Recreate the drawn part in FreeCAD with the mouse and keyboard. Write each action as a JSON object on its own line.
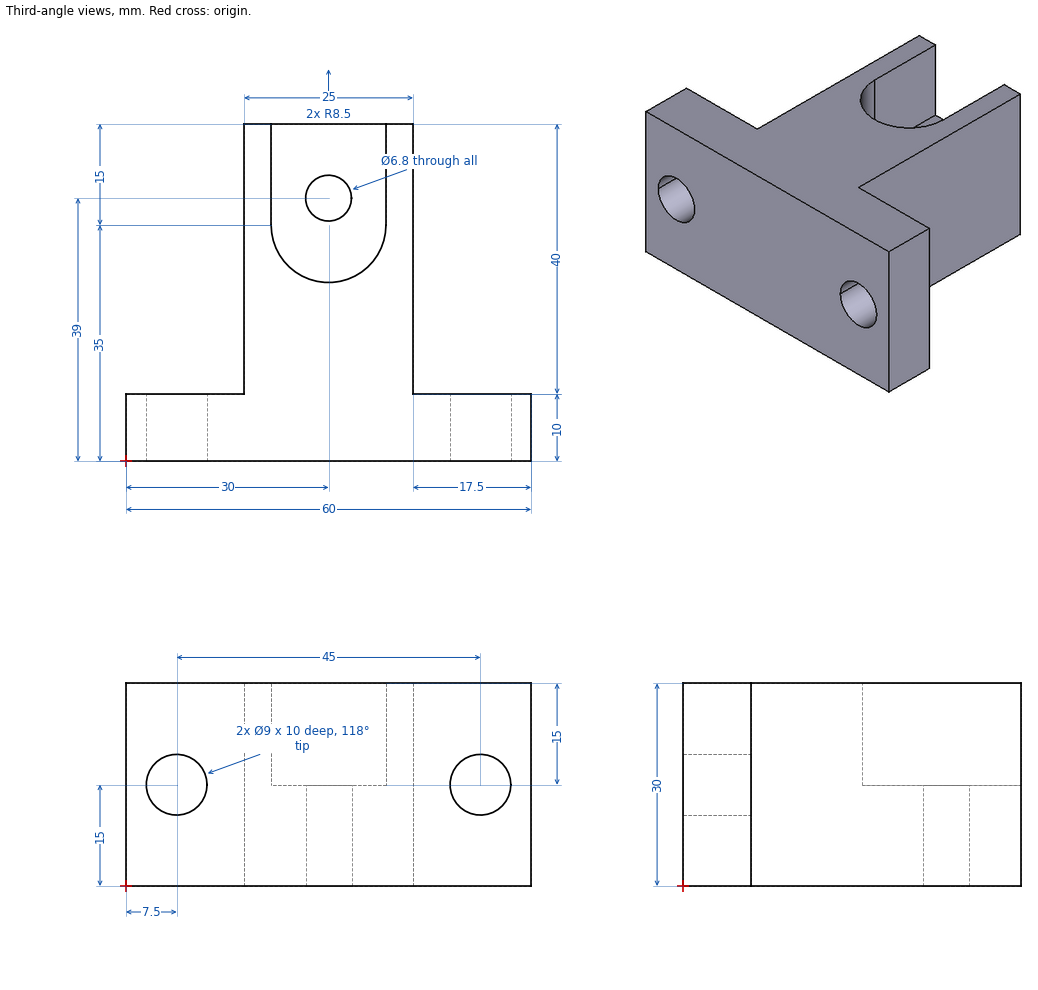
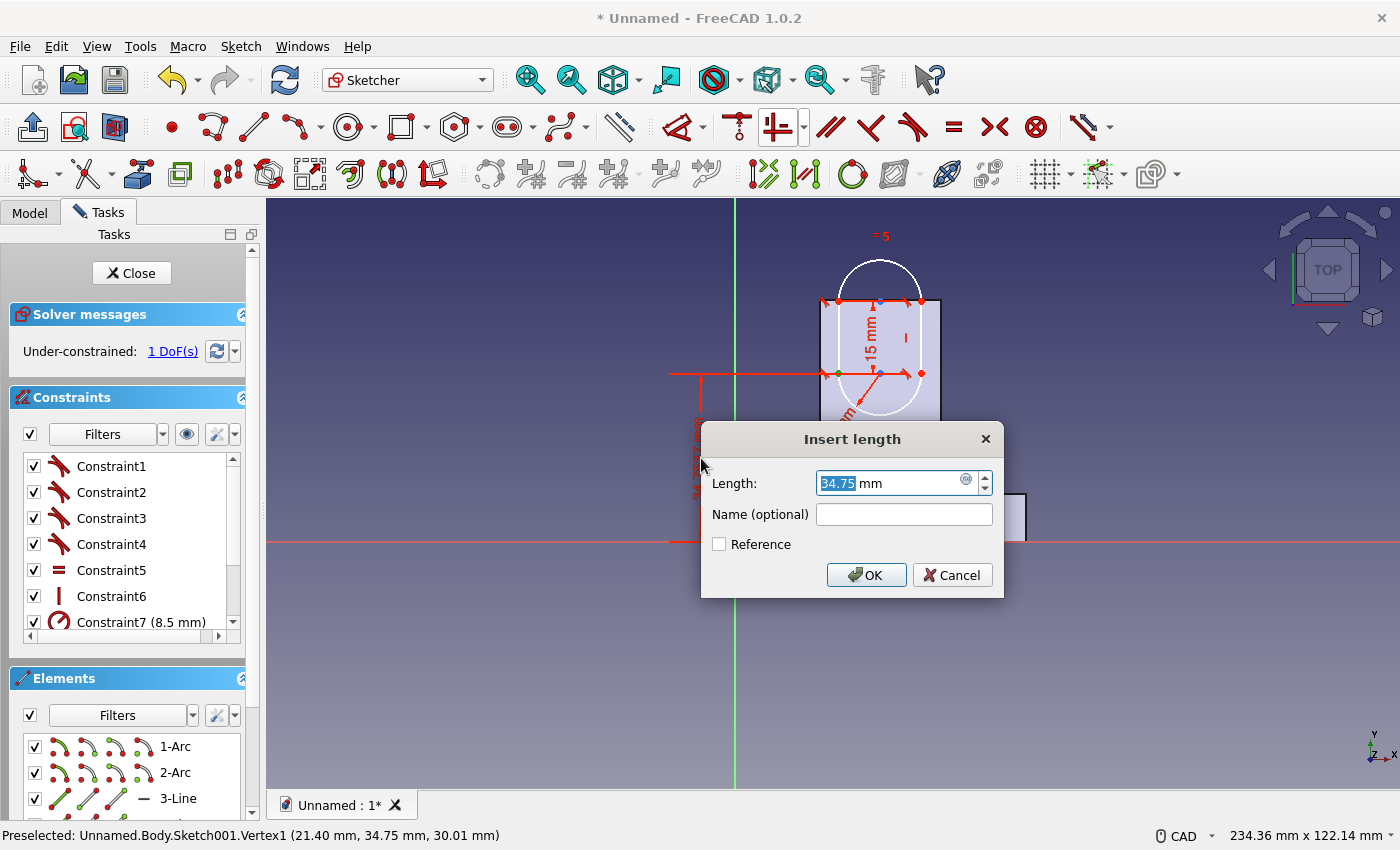
{"action": "type", "text": "35"}
{"action": "key", "text": "Return"}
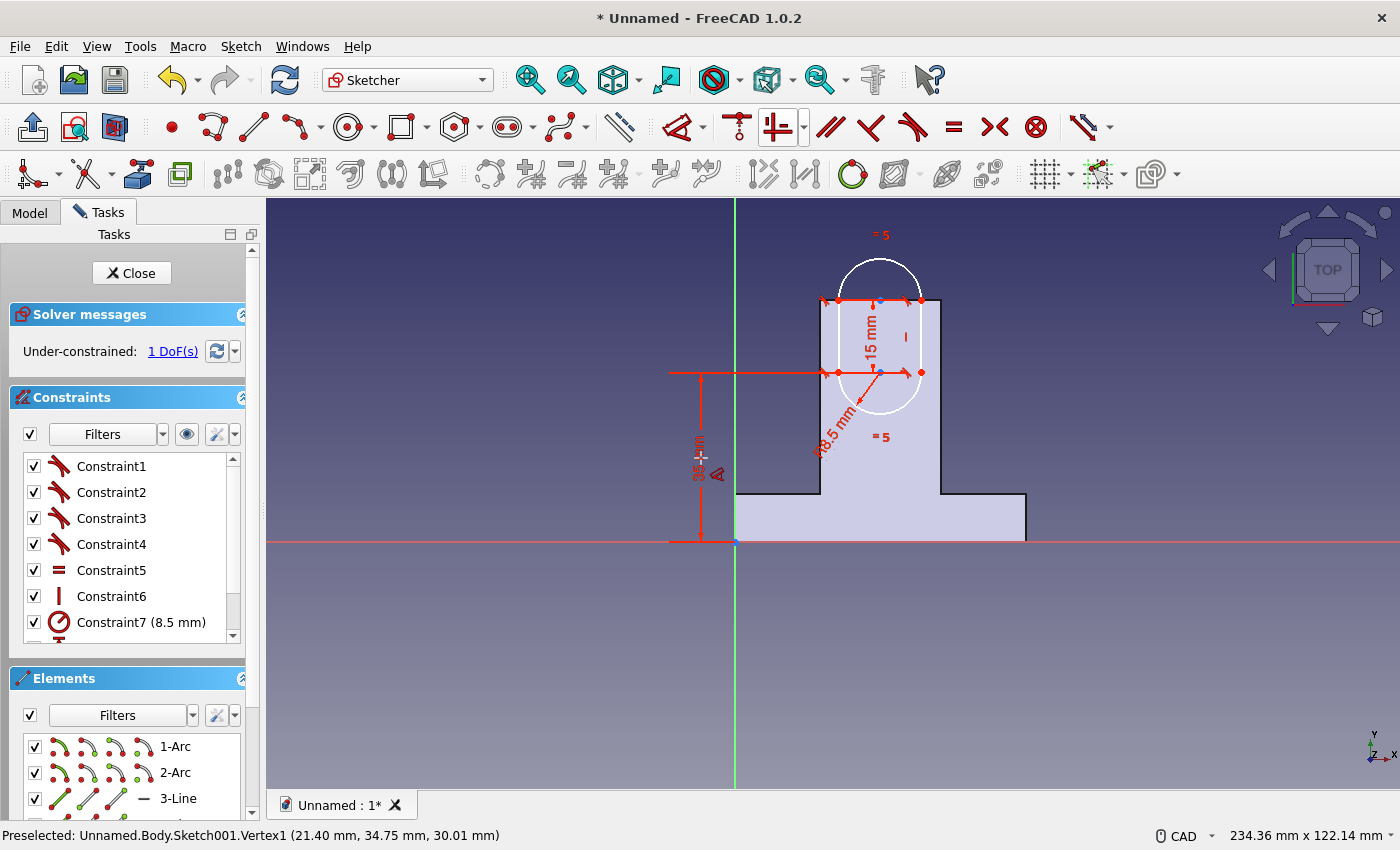
{"action": "left_click", "coordinate": [880, 373]}
{"action": "left_click", "coordinate": [808, 576]}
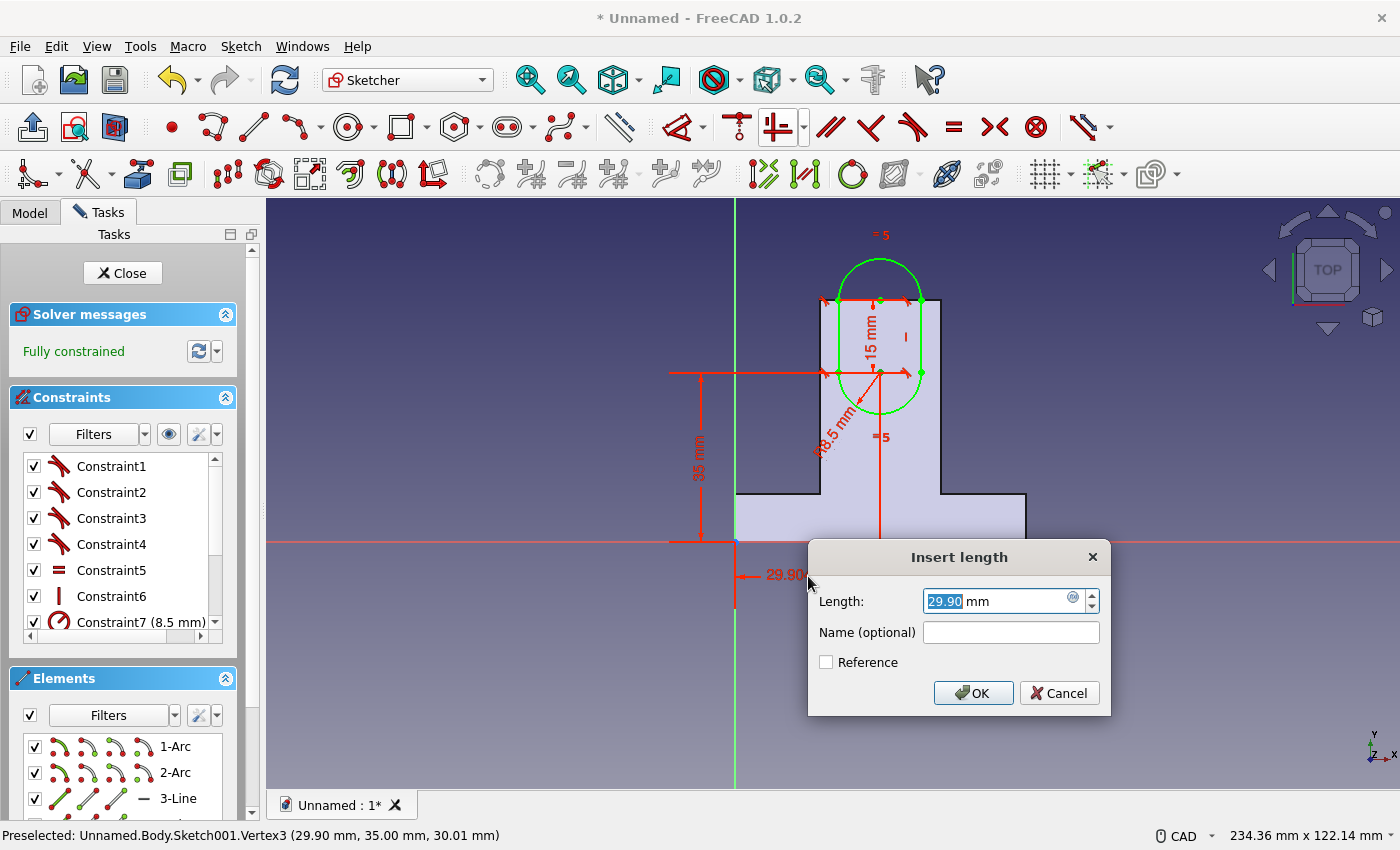
{"action": "type", "text": "30"}
{"action": "key", "text": "Return"}
{"action": "key", "text": "Escape"}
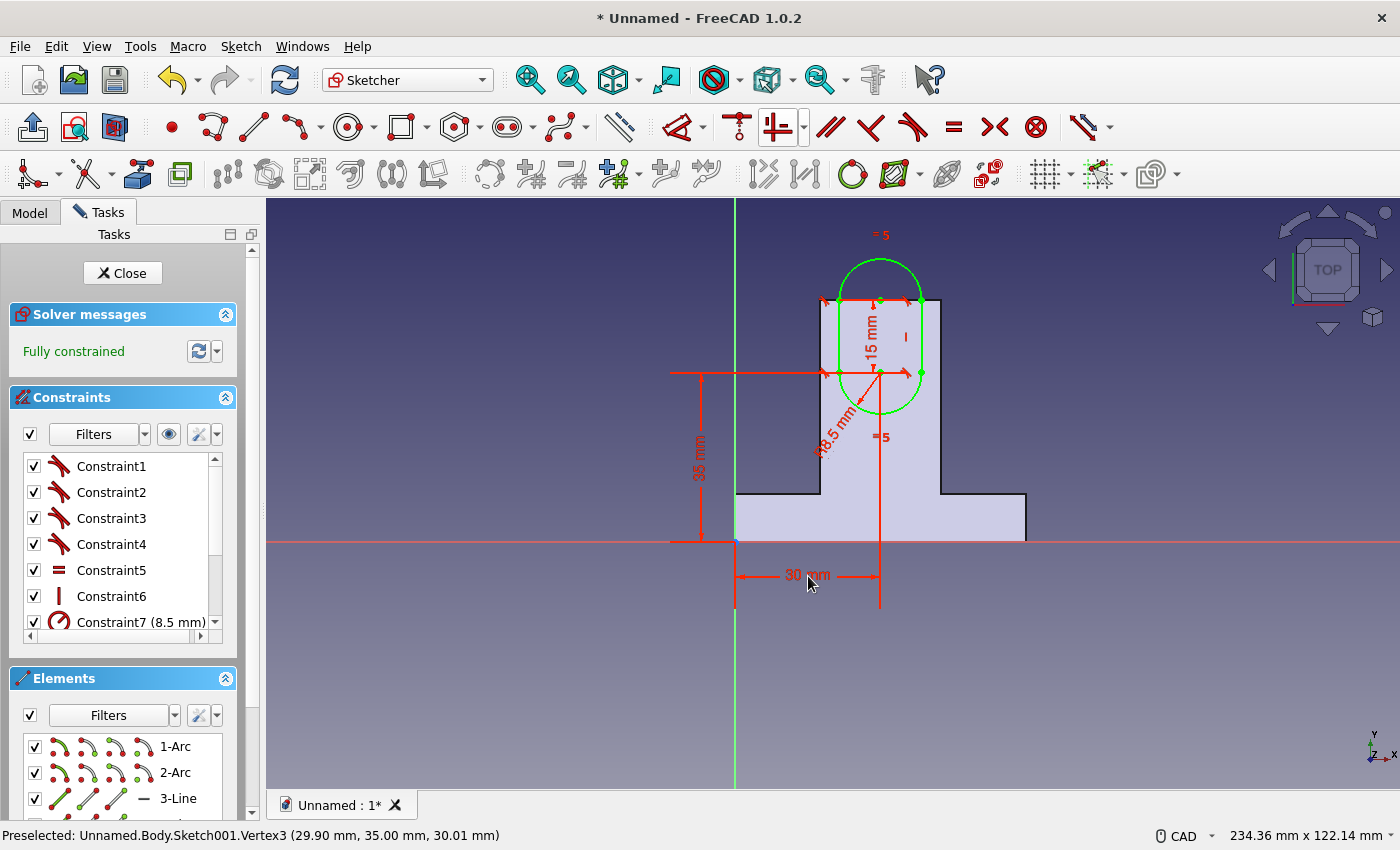
{"action": "left_click", "coordinate": [123, 273]}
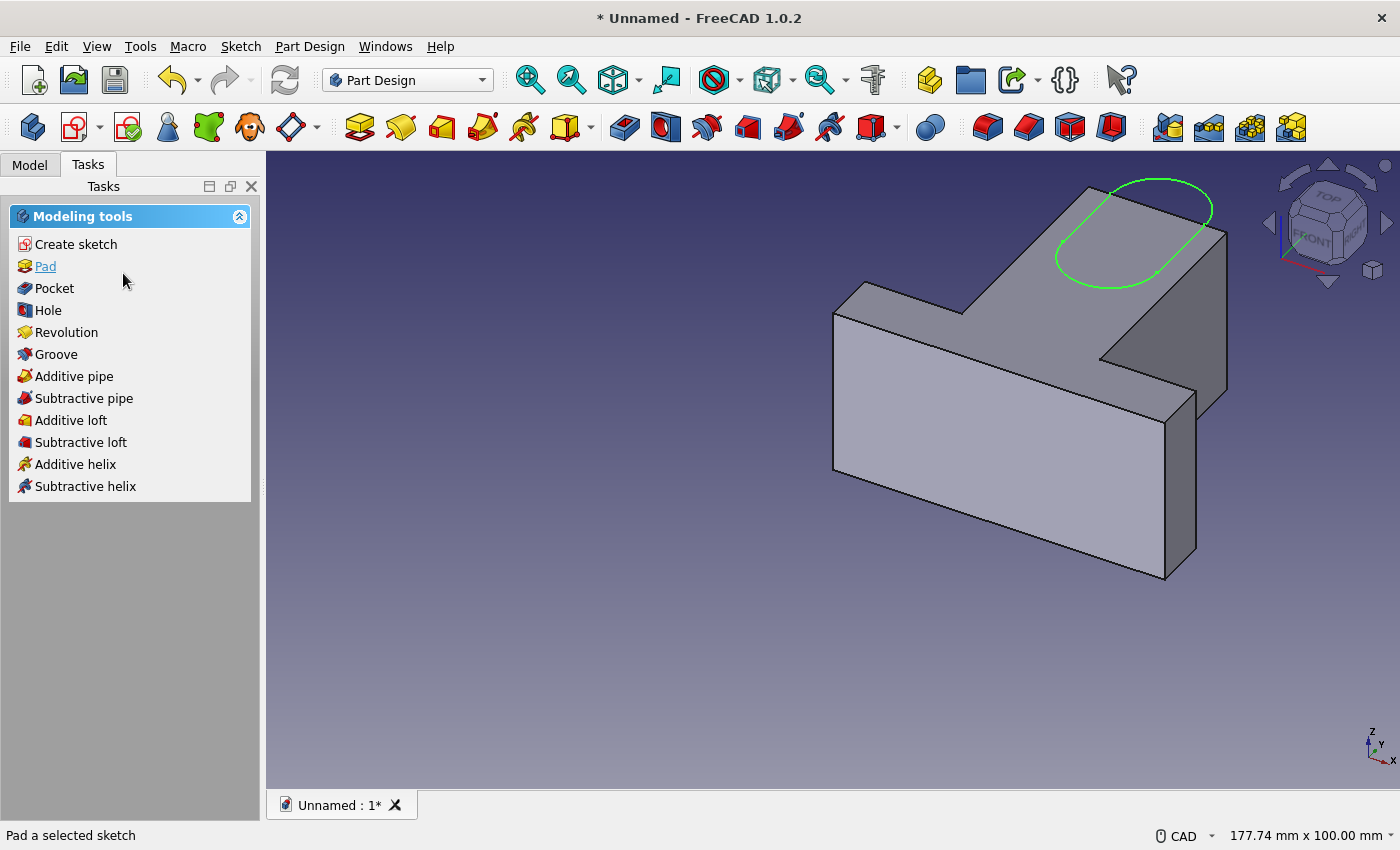
{"action": "left_click", "coordinate": [625, 128]}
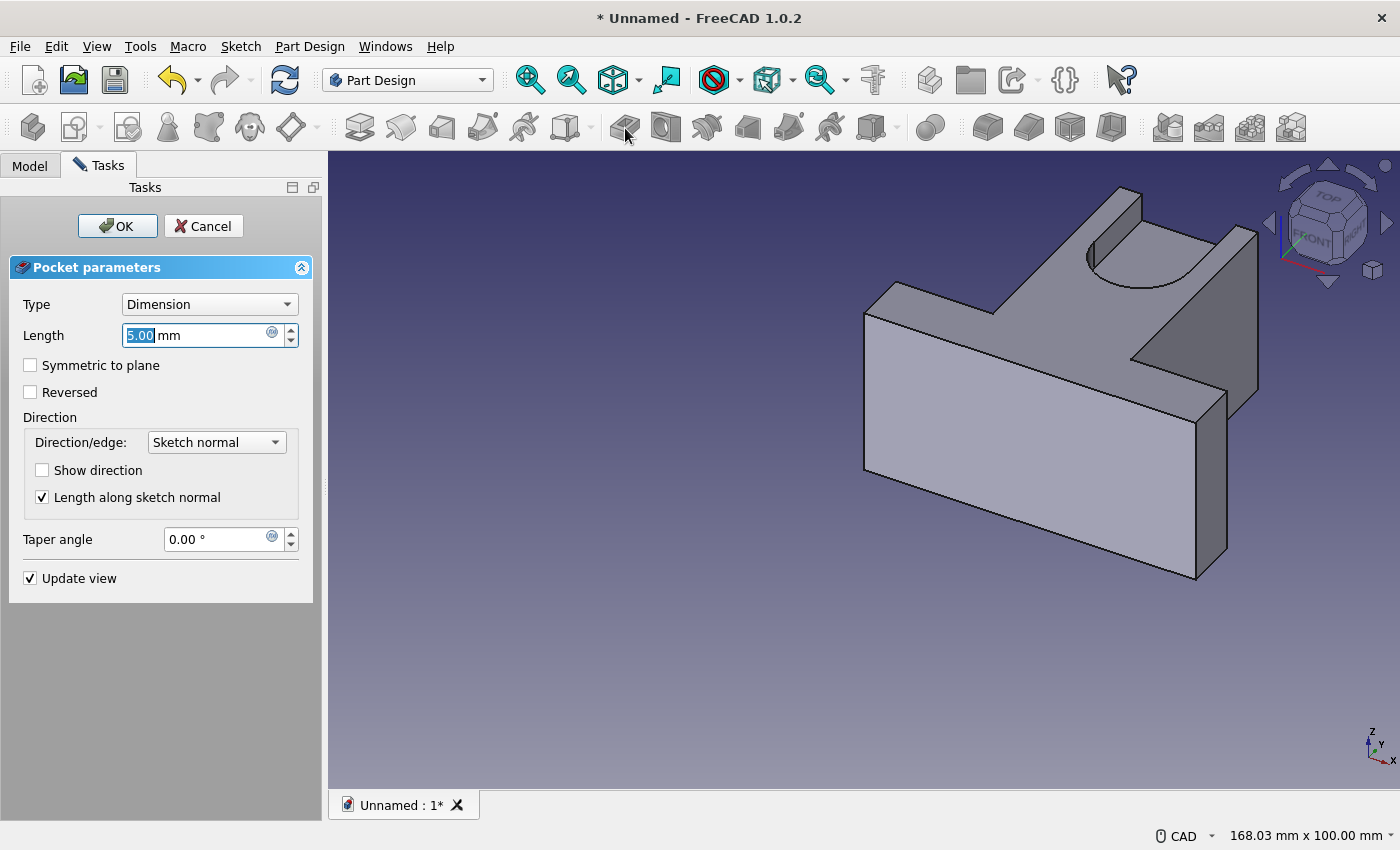
{"action": "type", "text": "15"}
{"action": "key", "text": "Tab"}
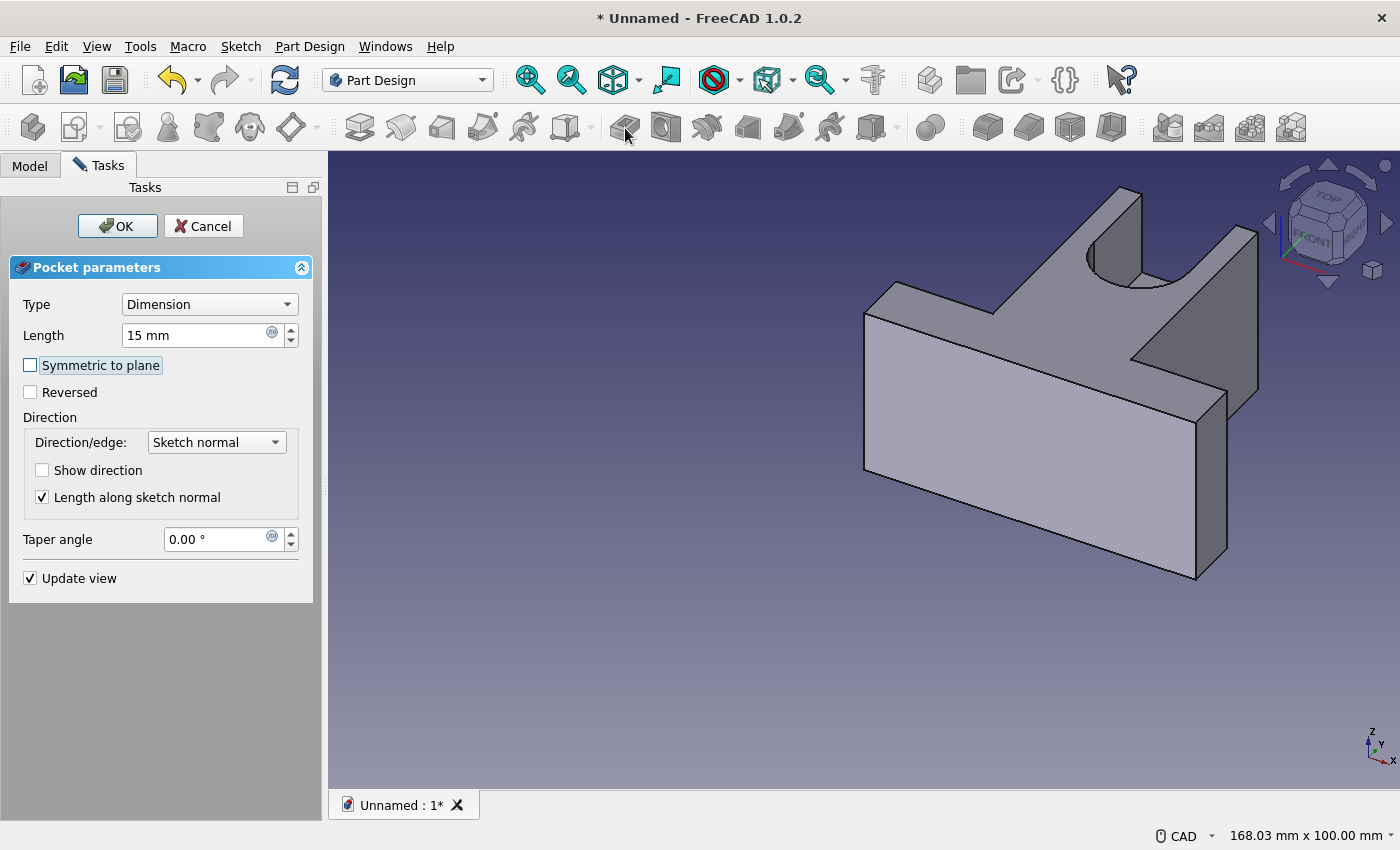
{"action": "left_click", "coordinate": [118, 226]}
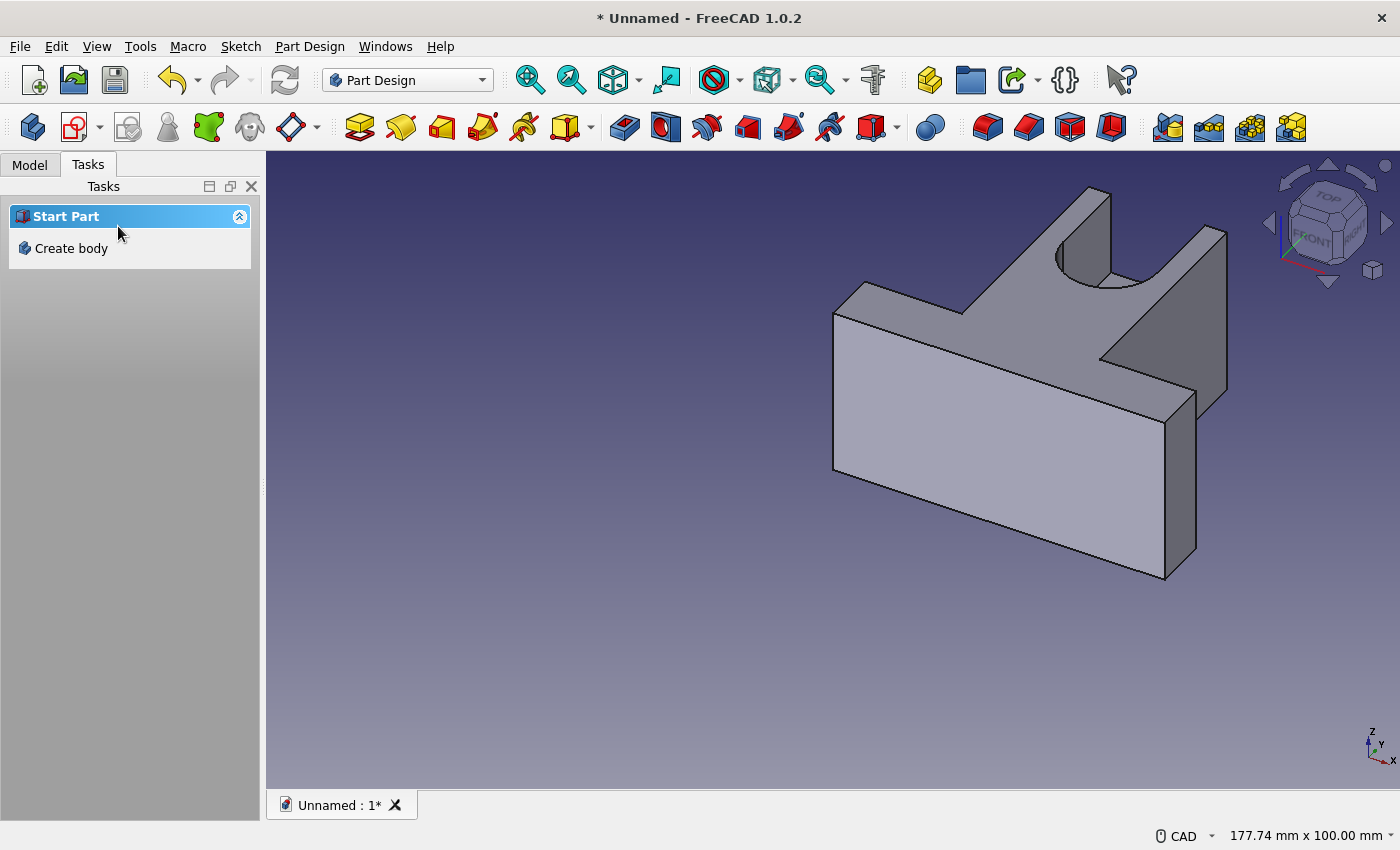
{"action": "left_click", "coordinate": [1046, 461]}